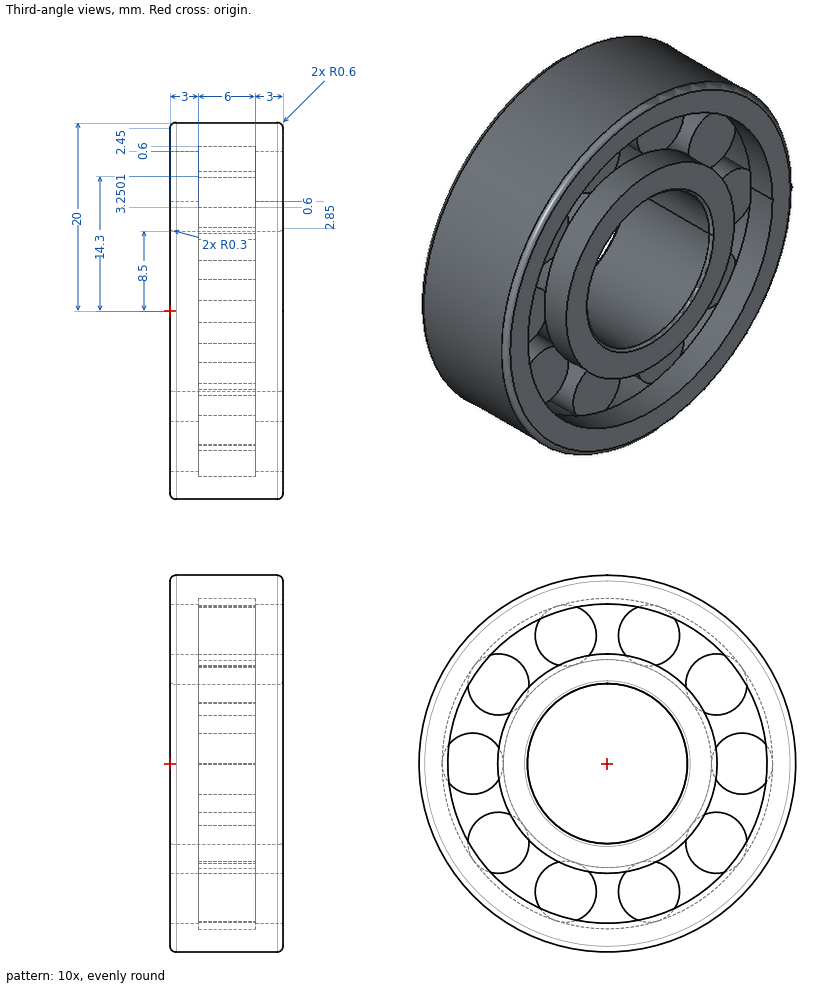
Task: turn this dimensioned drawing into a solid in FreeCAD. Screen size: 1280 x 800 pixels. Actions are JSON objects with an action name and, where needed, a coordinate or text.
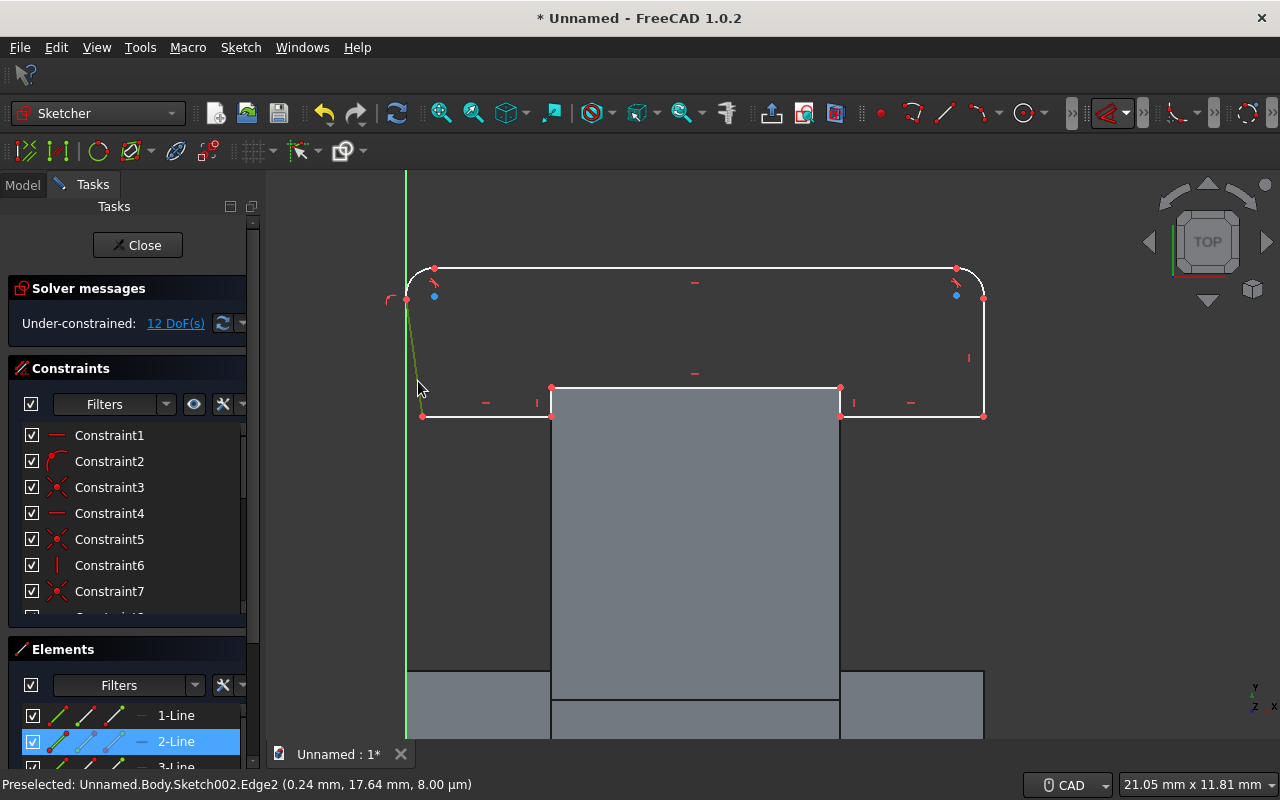
{"action": "left_click", "coordinate": [420, 272]}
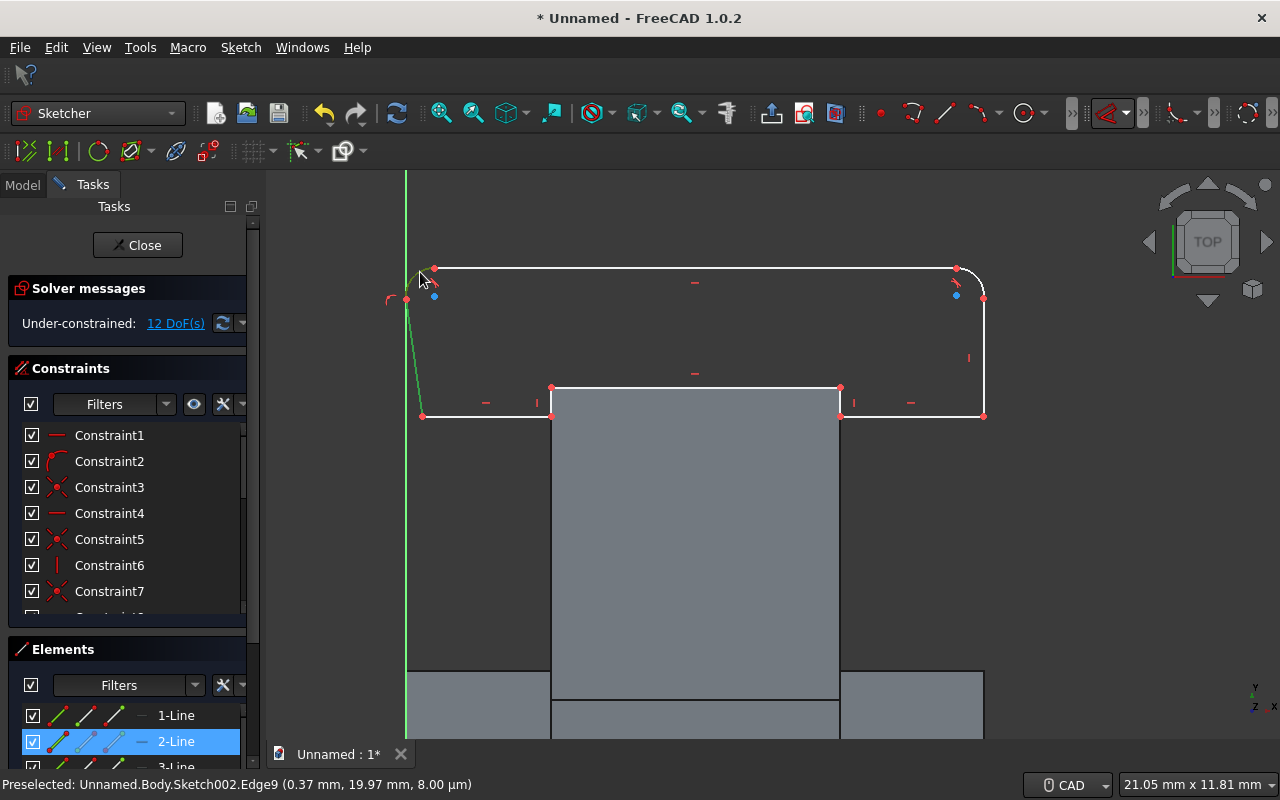
{"action": "key", "text": "t"}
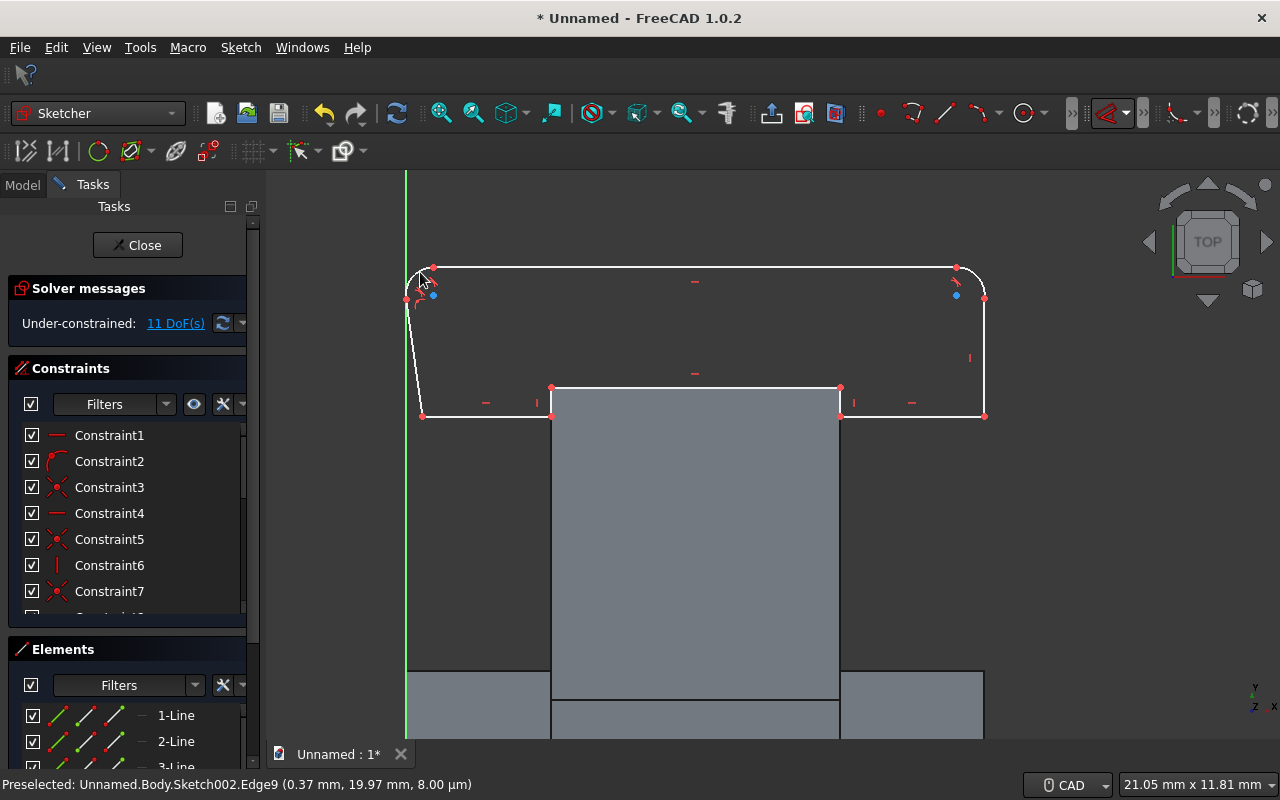
{"action": "left_click", "coordinate": [984, 381]}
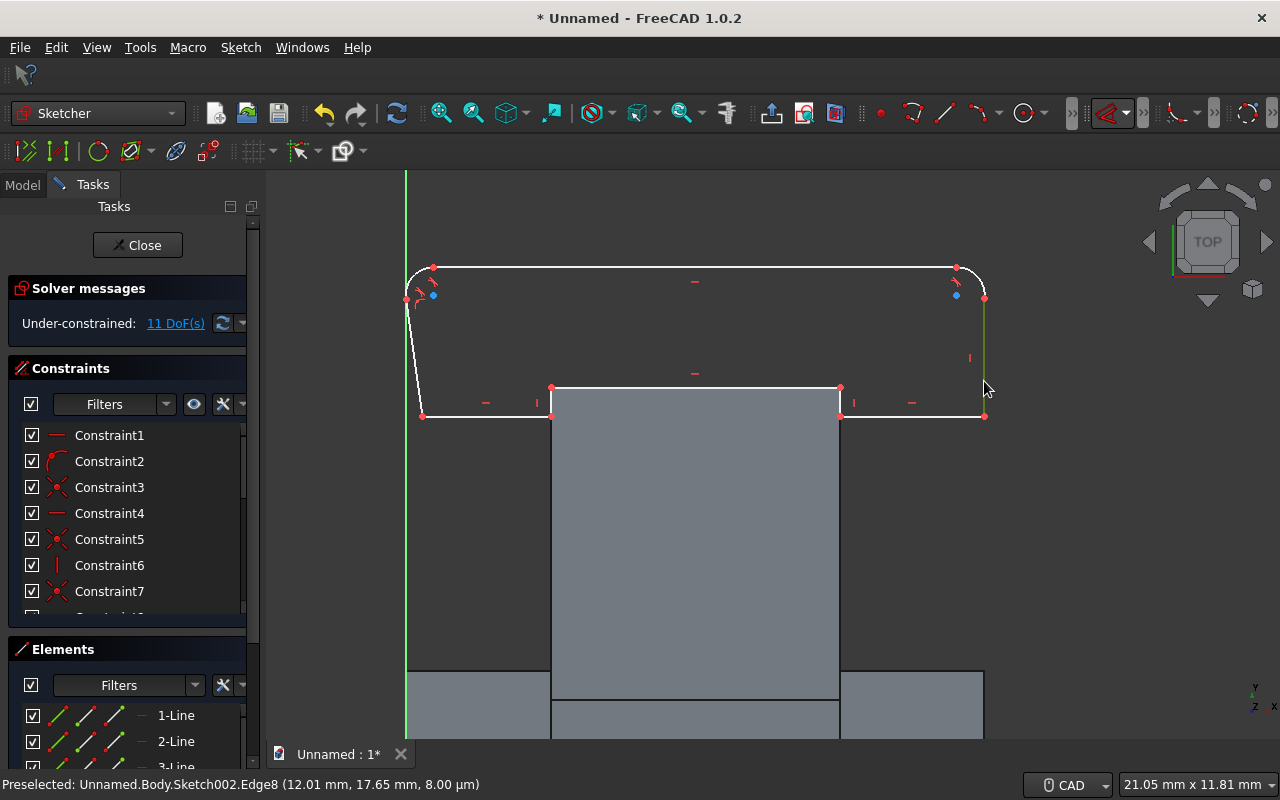
{"action": "left_click", "coordinate": [983, 285]}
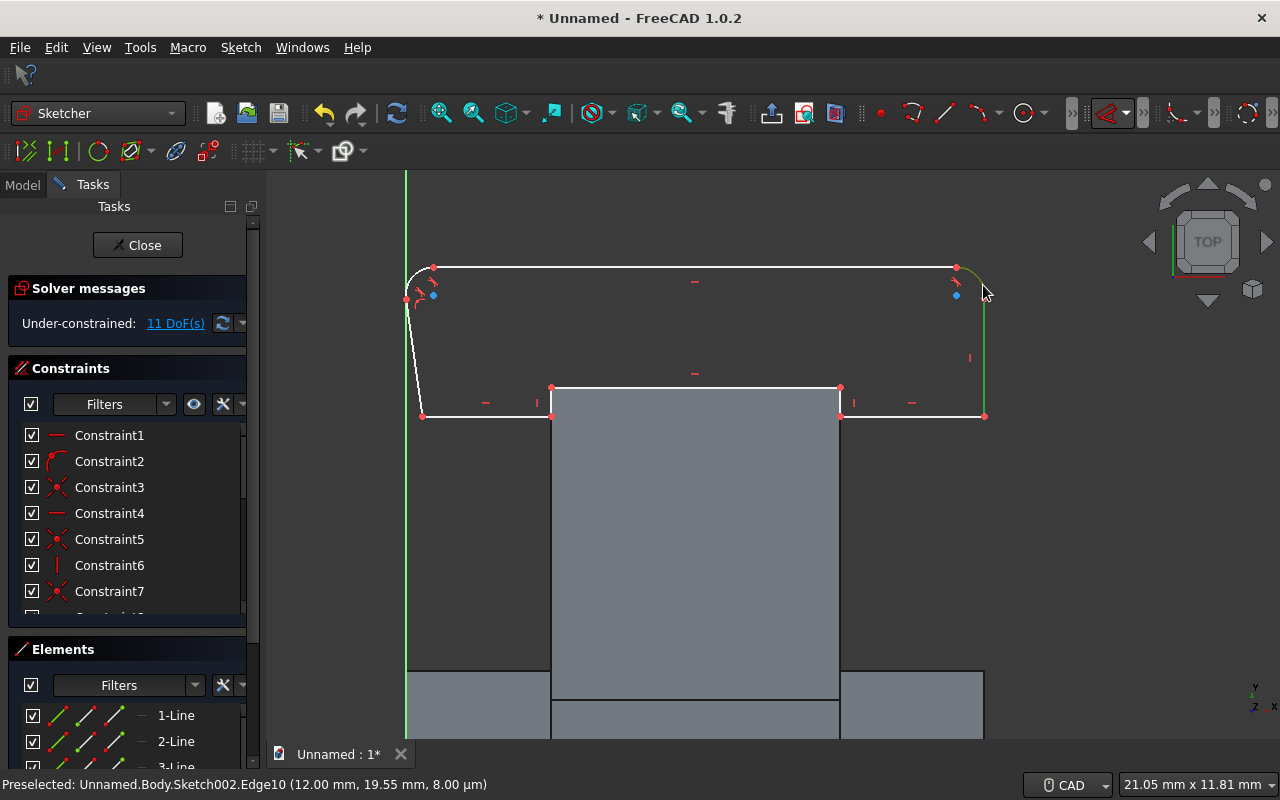
{"action": "key", "text": "t"}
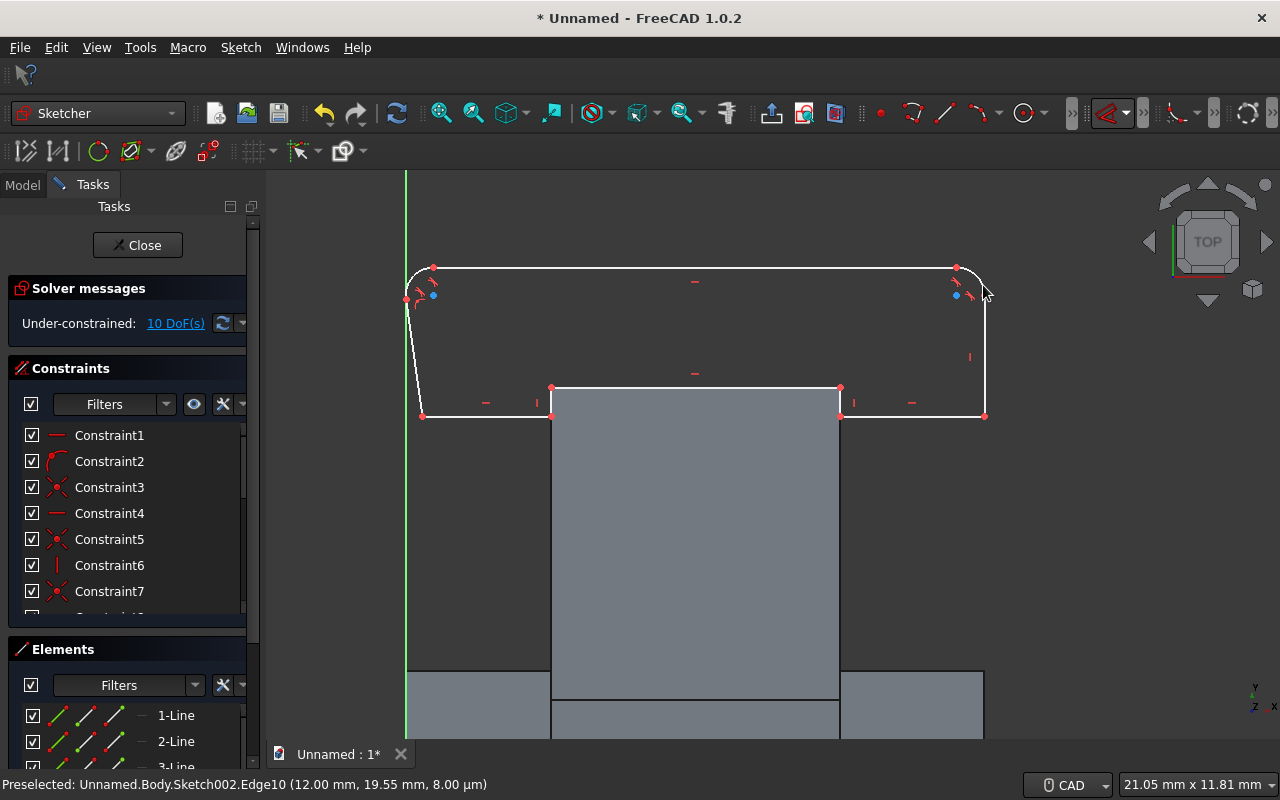
{"action": "left_click", "coordinate": [418, 381]}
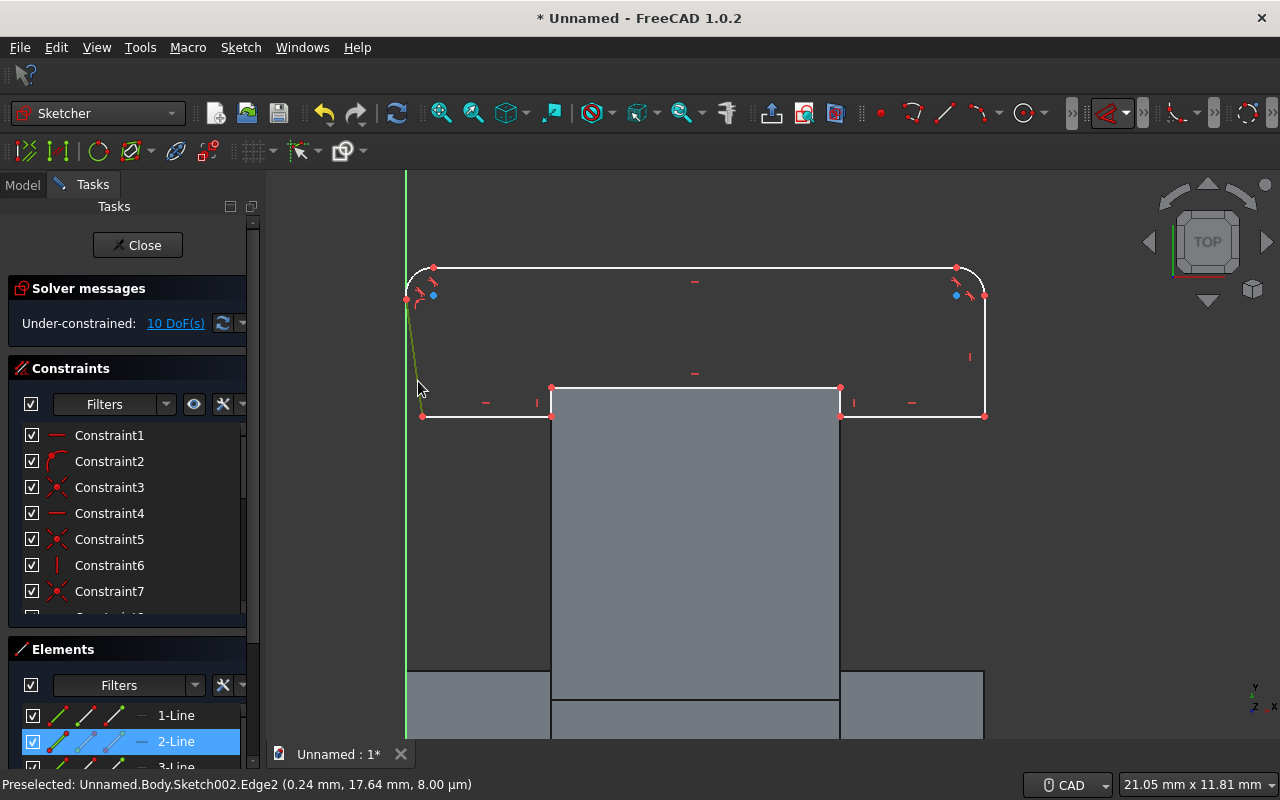
{"action": "key", "text": "v"}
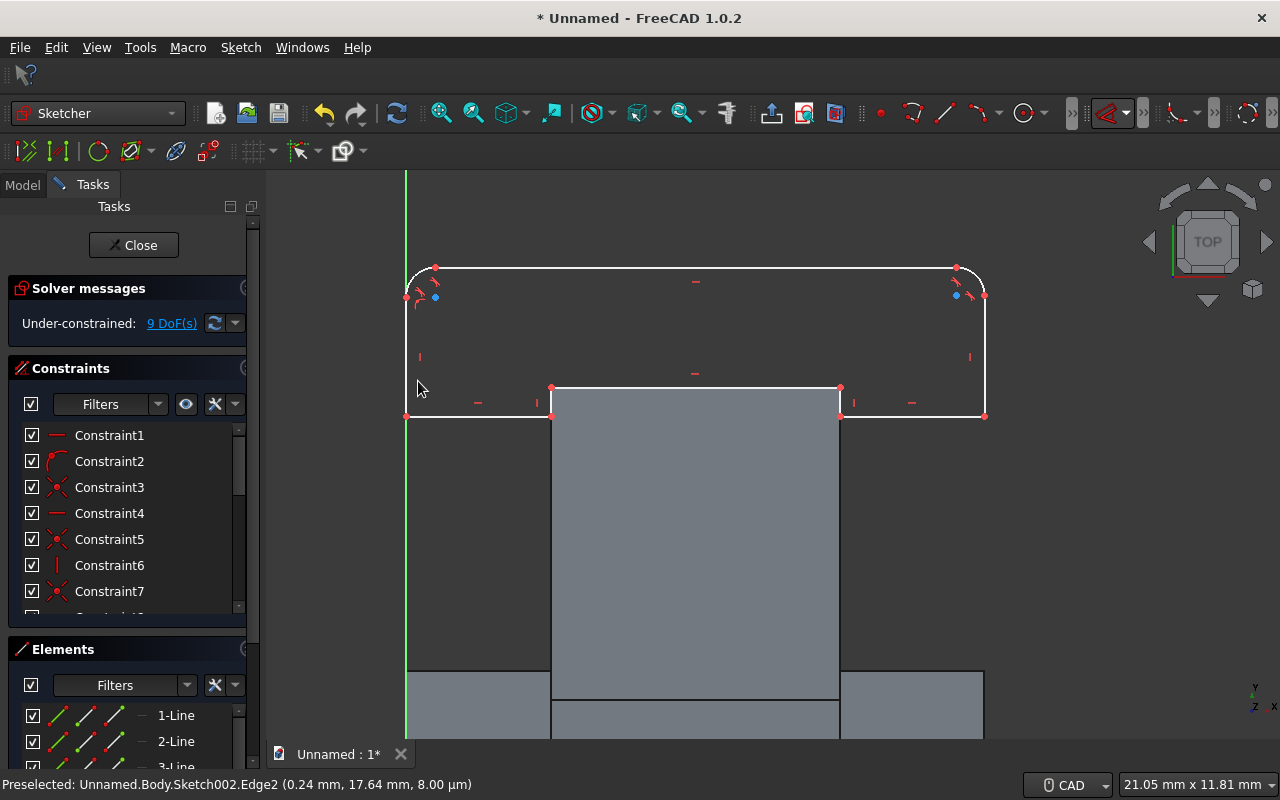
{"action": "left_click", "coordinate": [422, 271]}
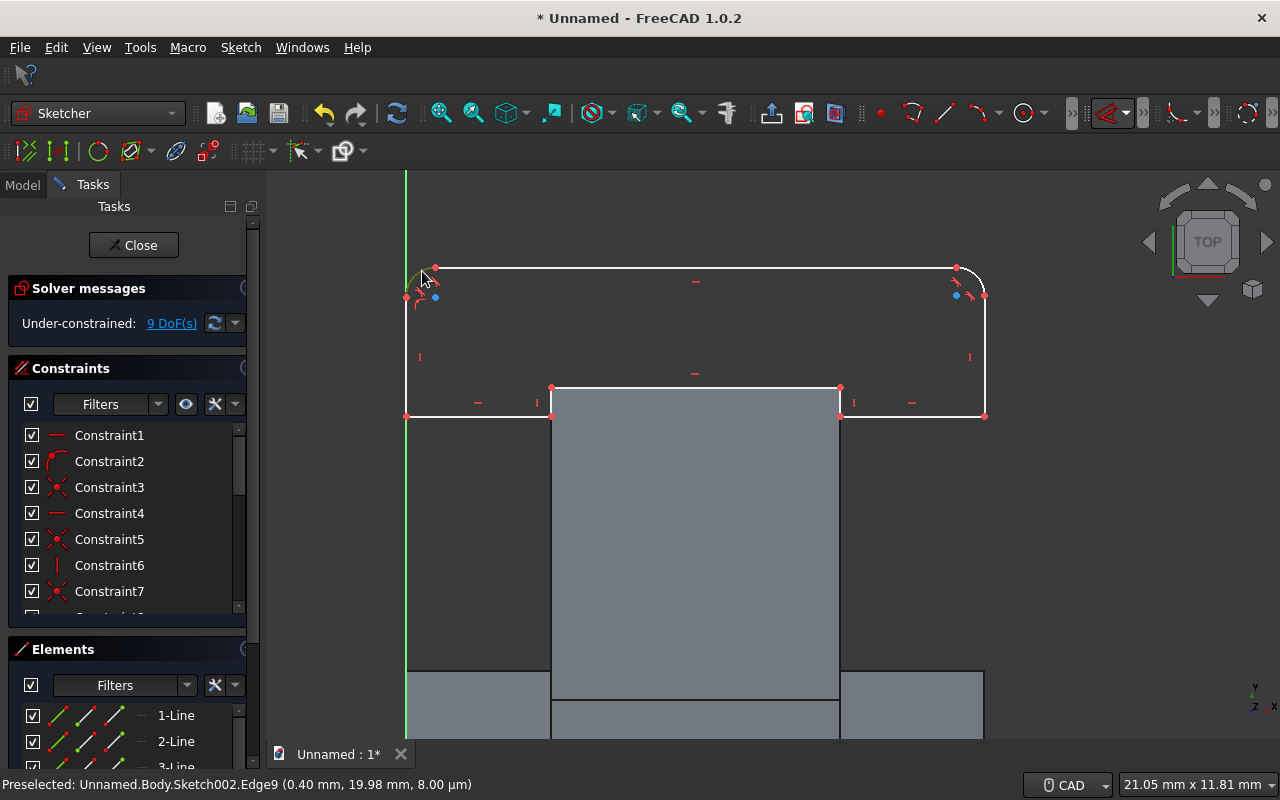
{"action": "left_click", "coordinate": [982, 283]}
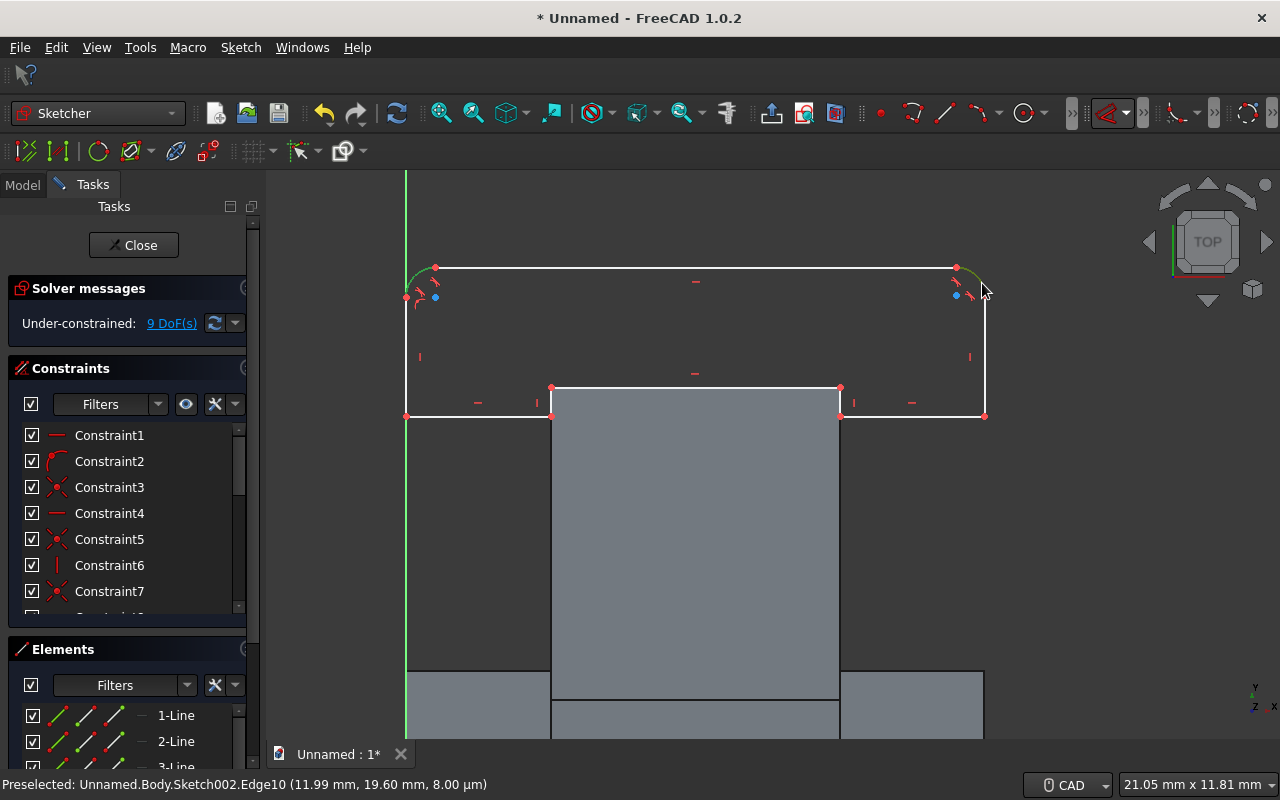
{"action": "key", "text": "e"}